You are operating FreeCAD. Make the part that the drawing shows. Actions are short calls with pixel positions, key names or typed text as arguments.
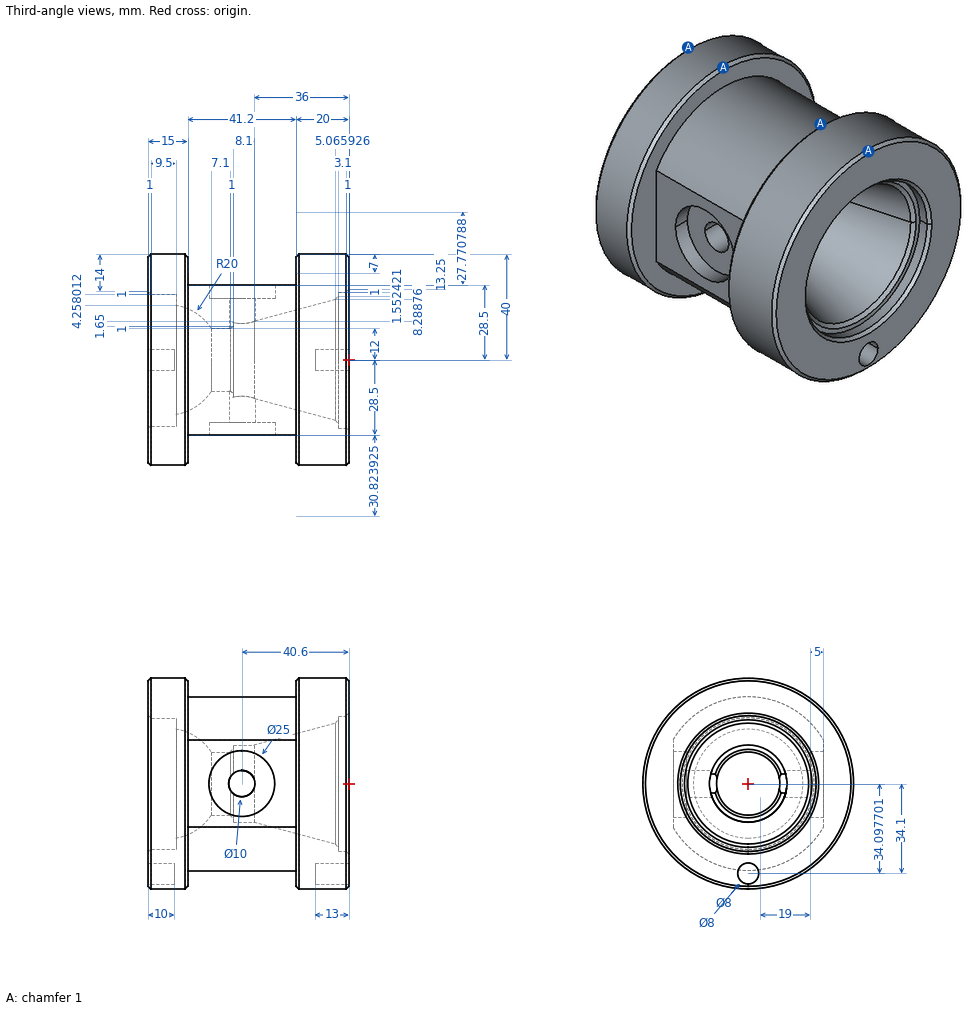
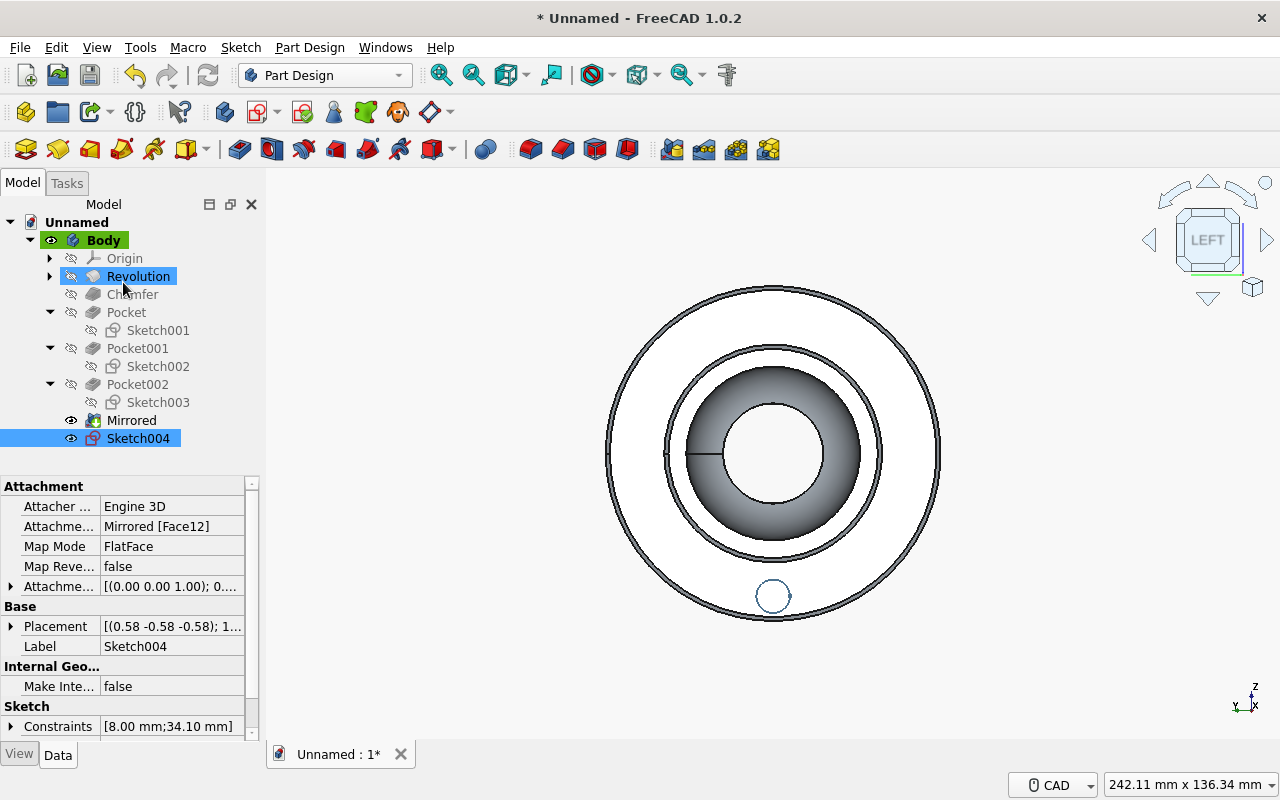
click(240, 150)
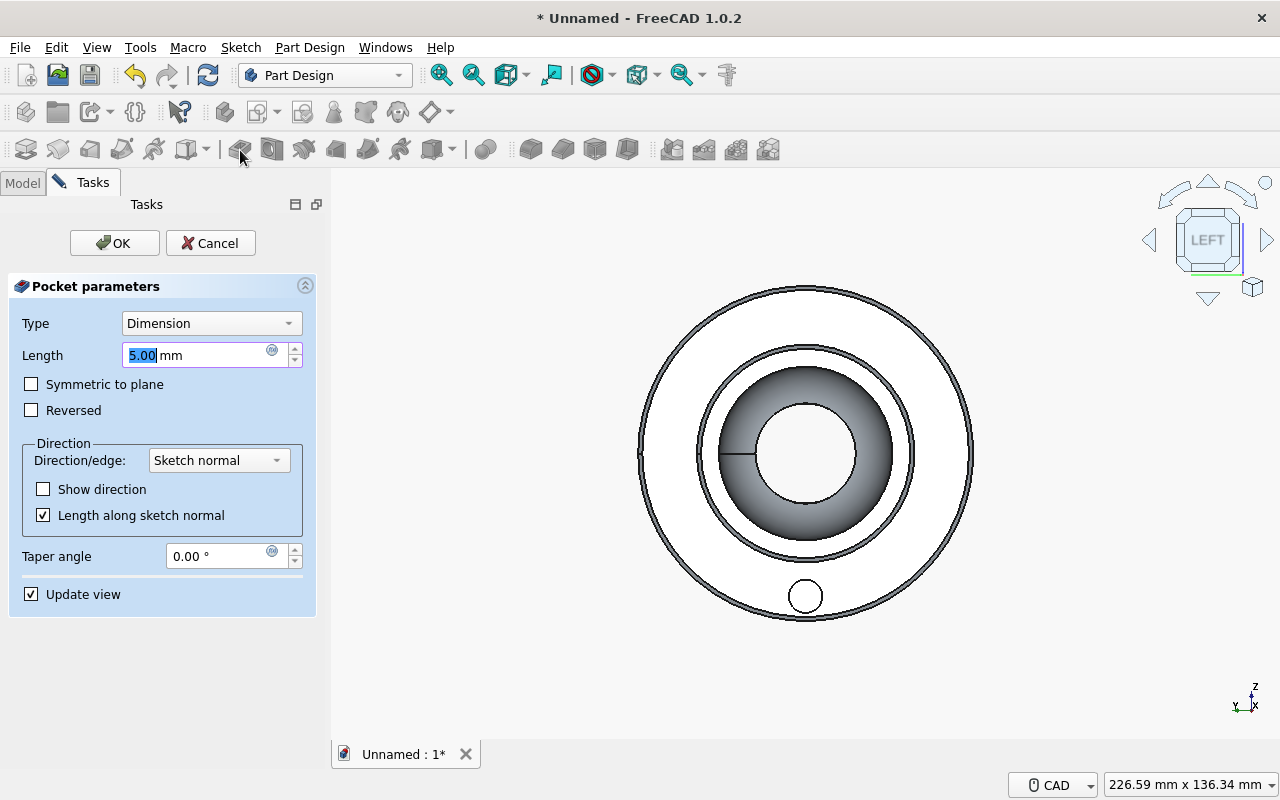
text(10)
key(Tab)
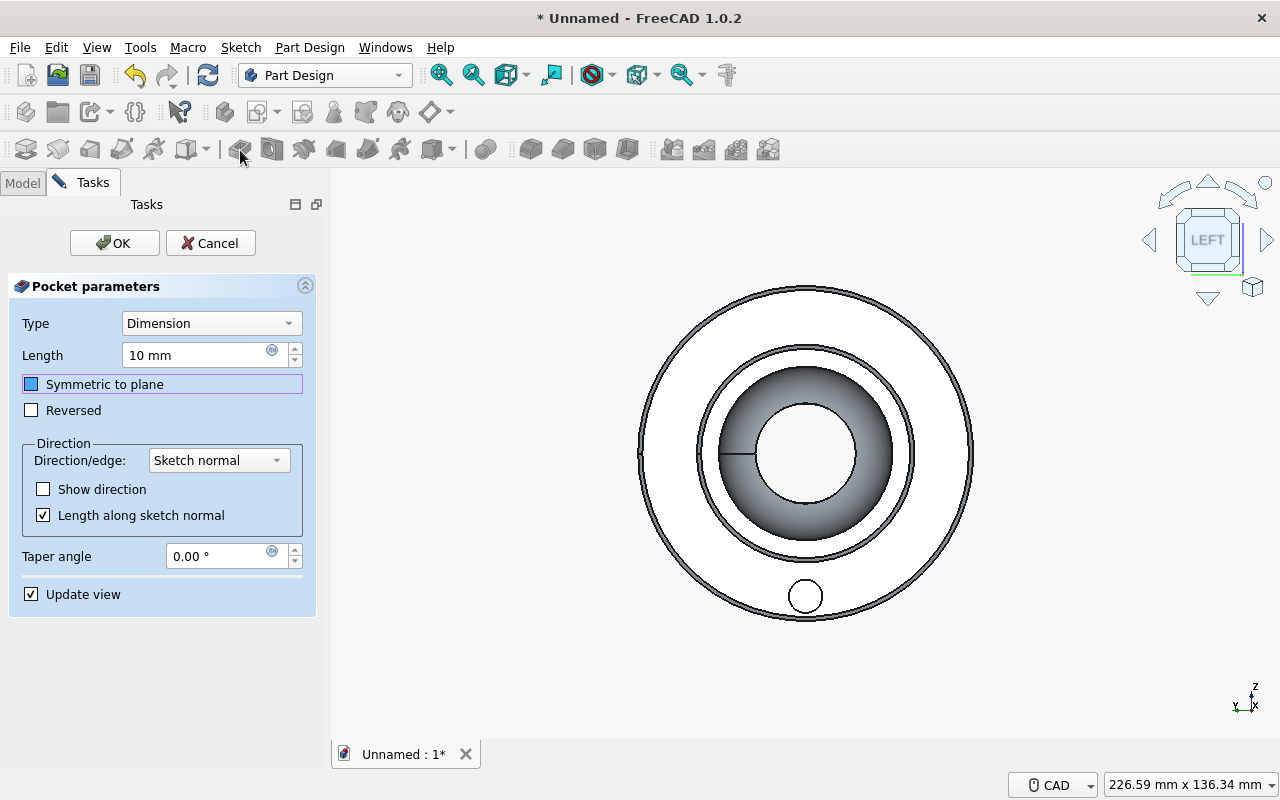
click(115, 243)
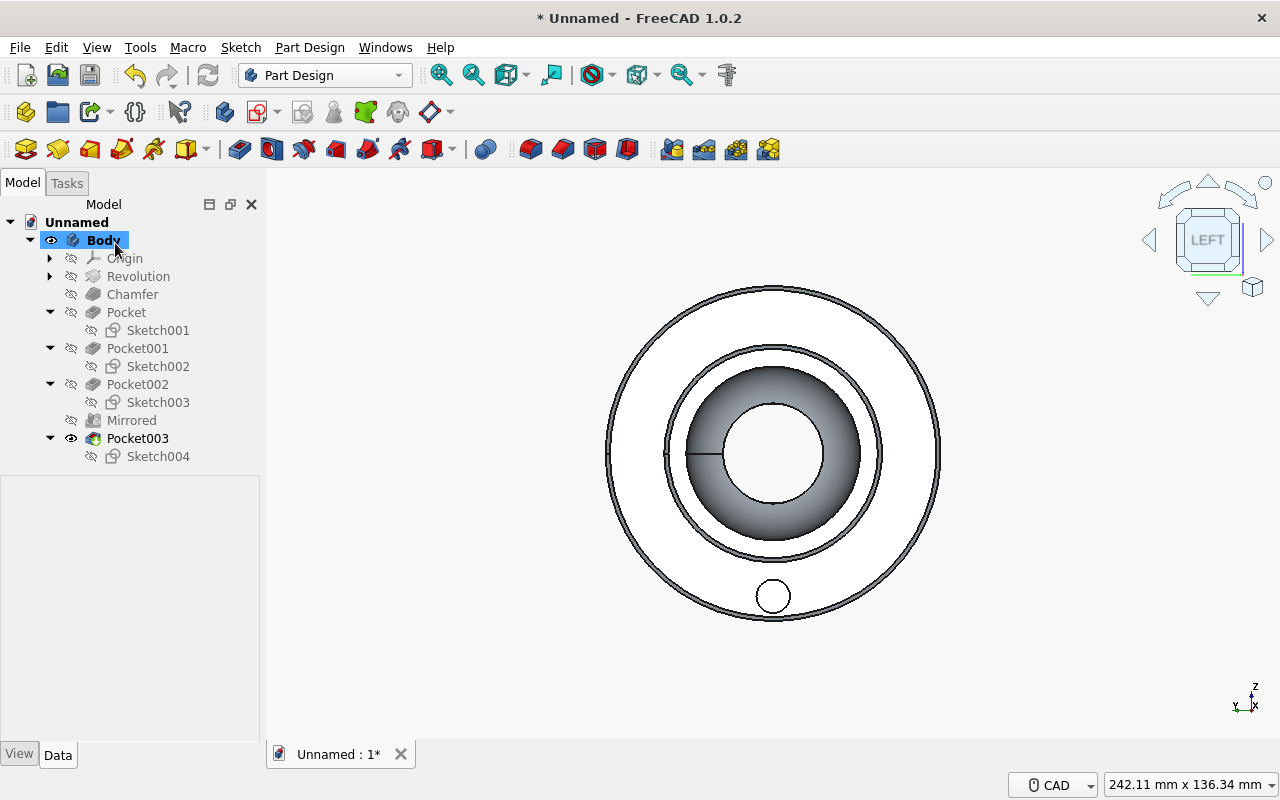
click(258, 112)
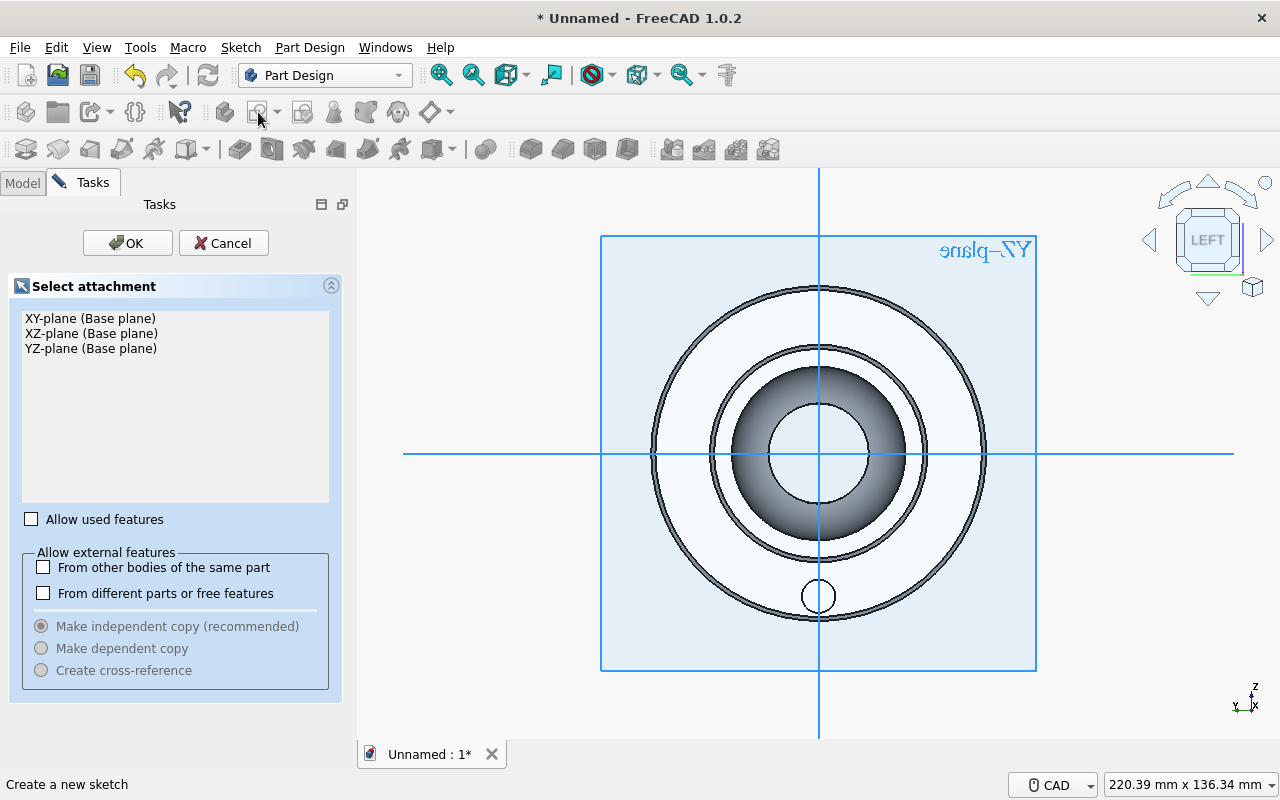
click(82, 348)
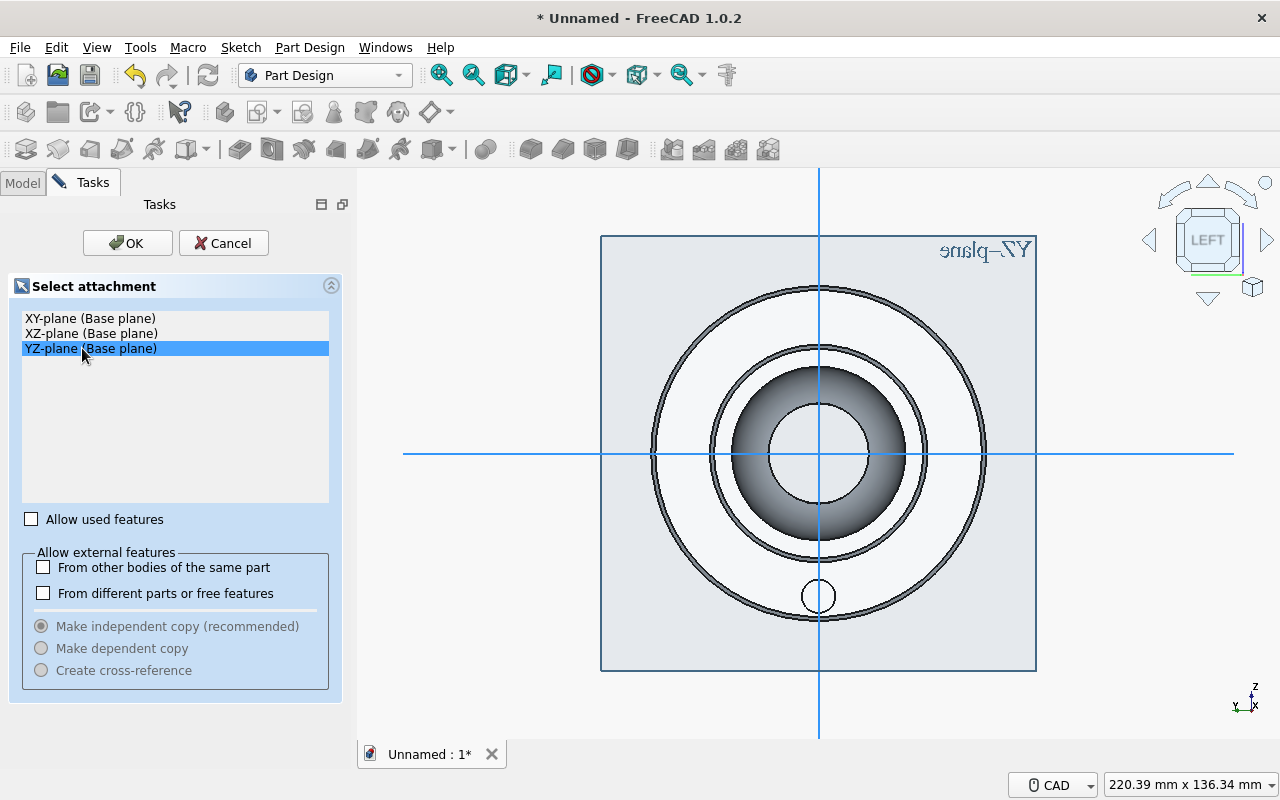
click(128, 243)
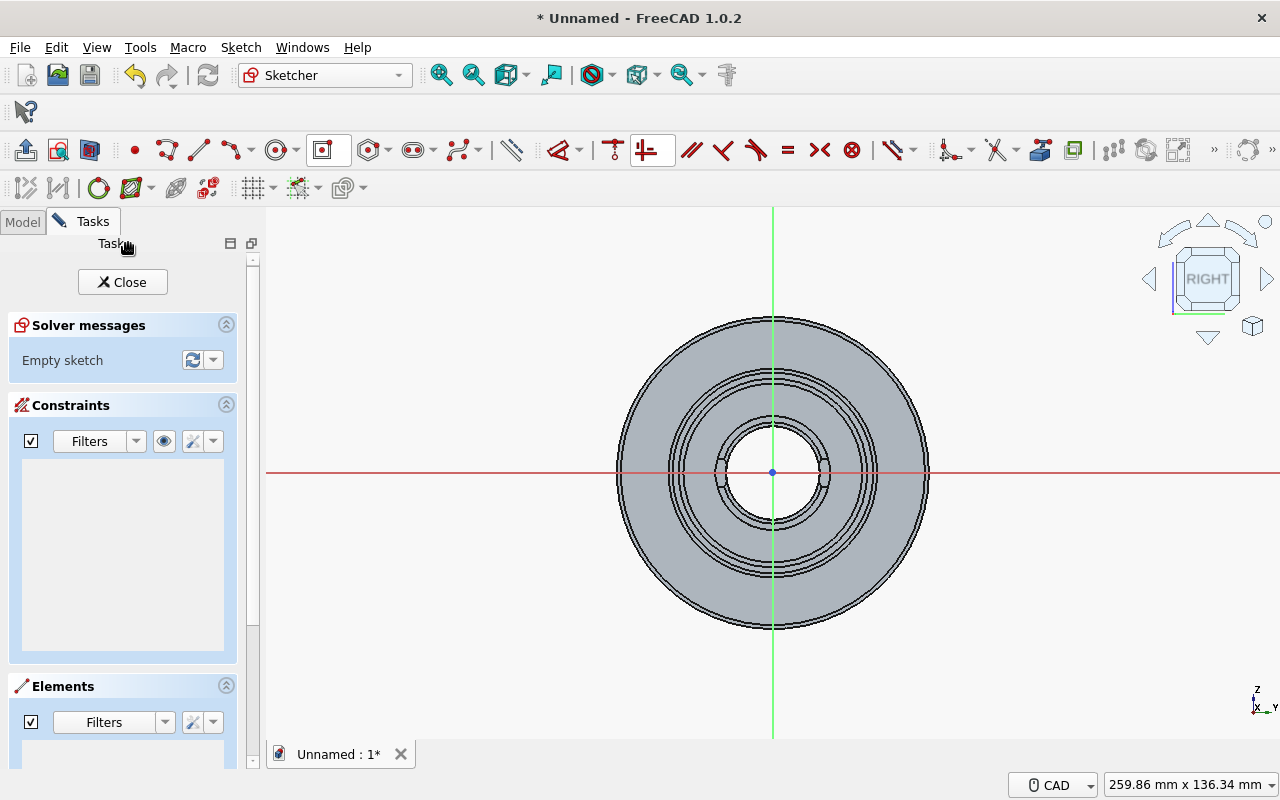
scroll(780, 619, up, 12)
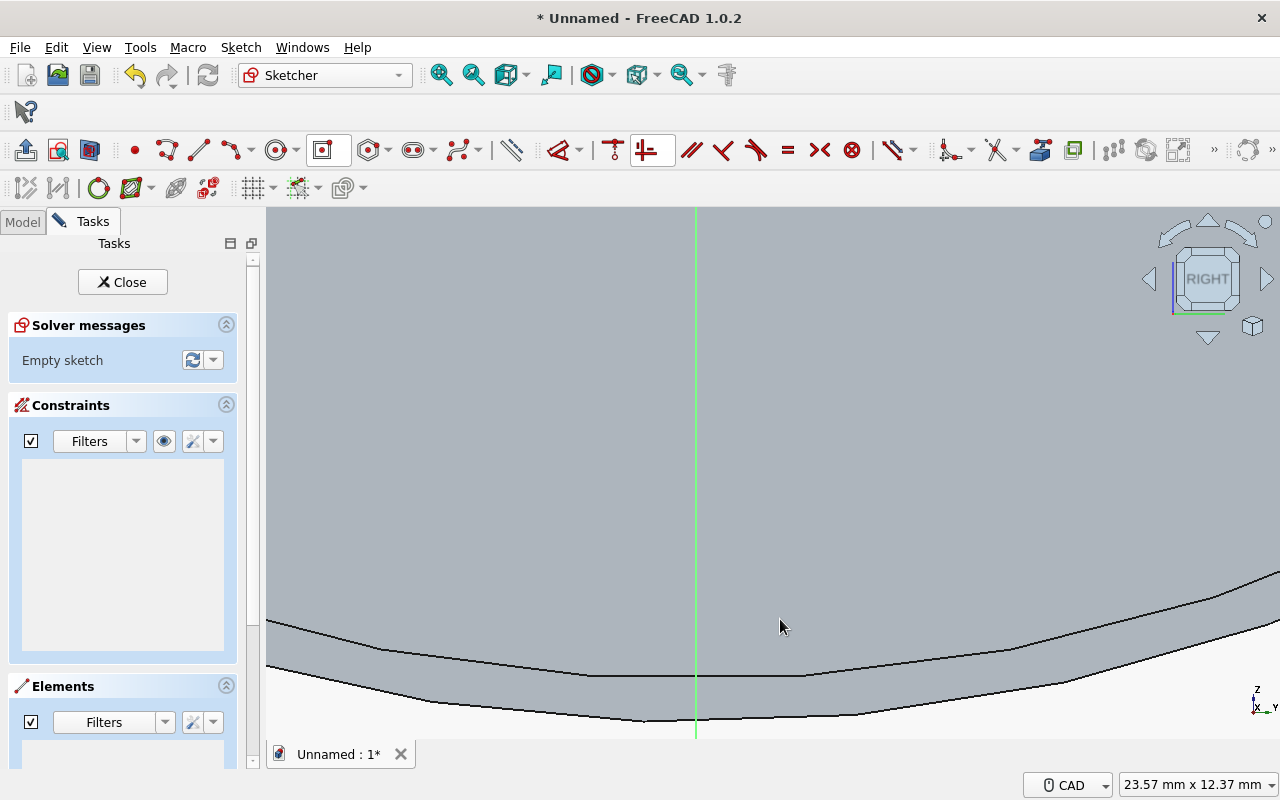
click(276, 150)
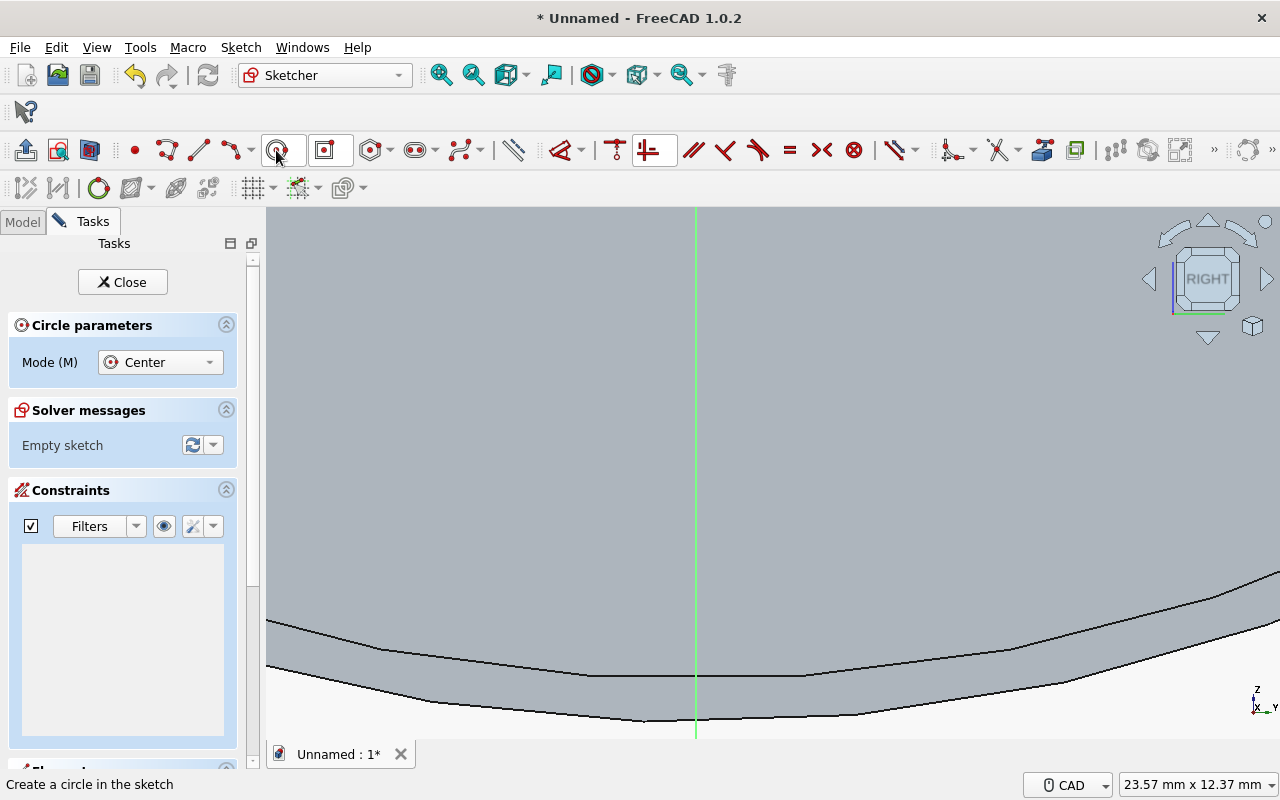
click(696, 469)
move(818, 347)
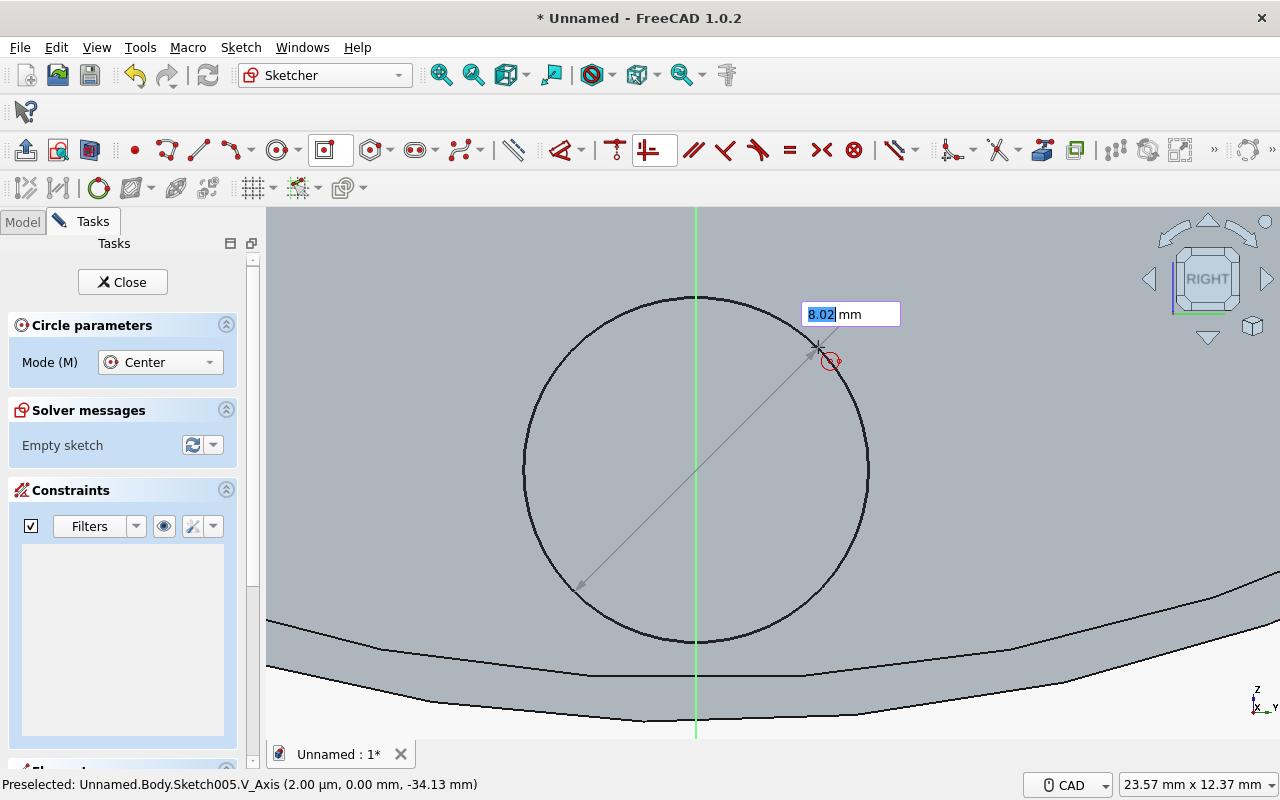
text(8)
key(Return)
key(Escape)